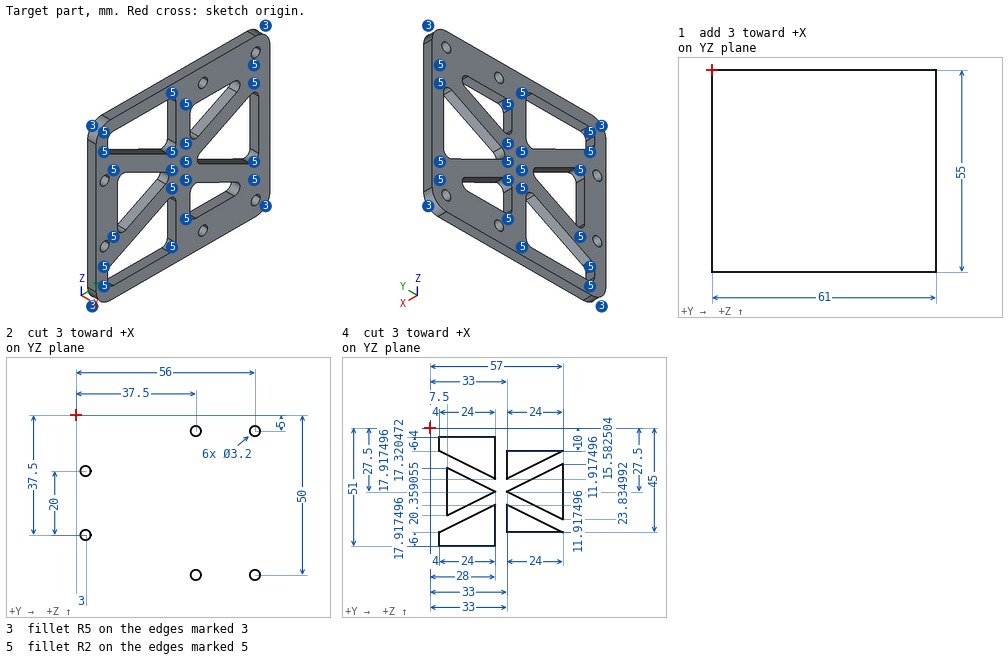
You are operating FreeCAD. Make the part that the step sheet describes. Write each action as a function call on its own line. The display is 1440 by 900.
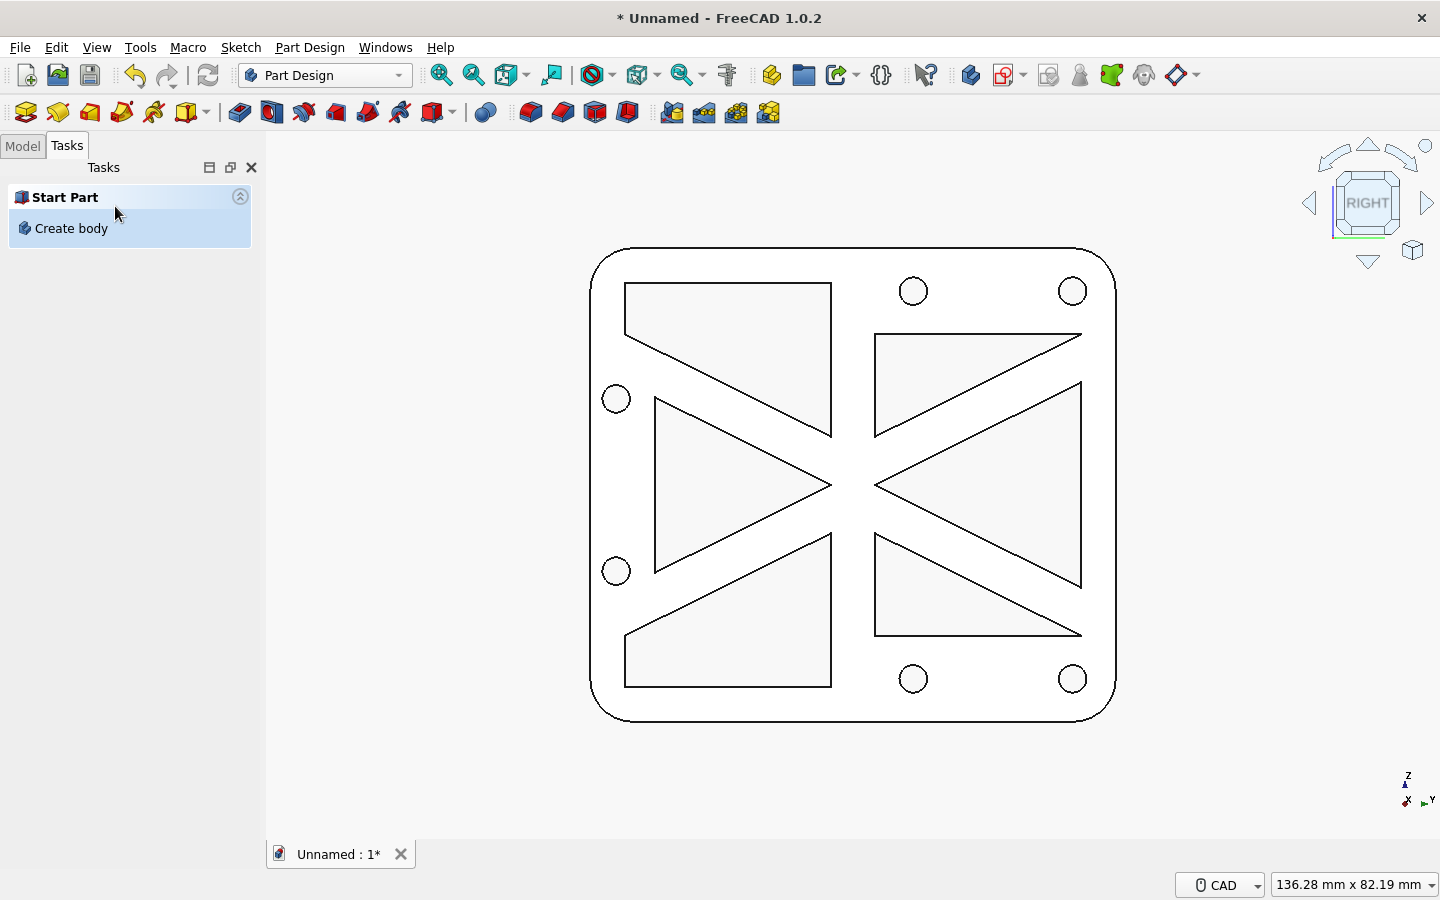
key(5)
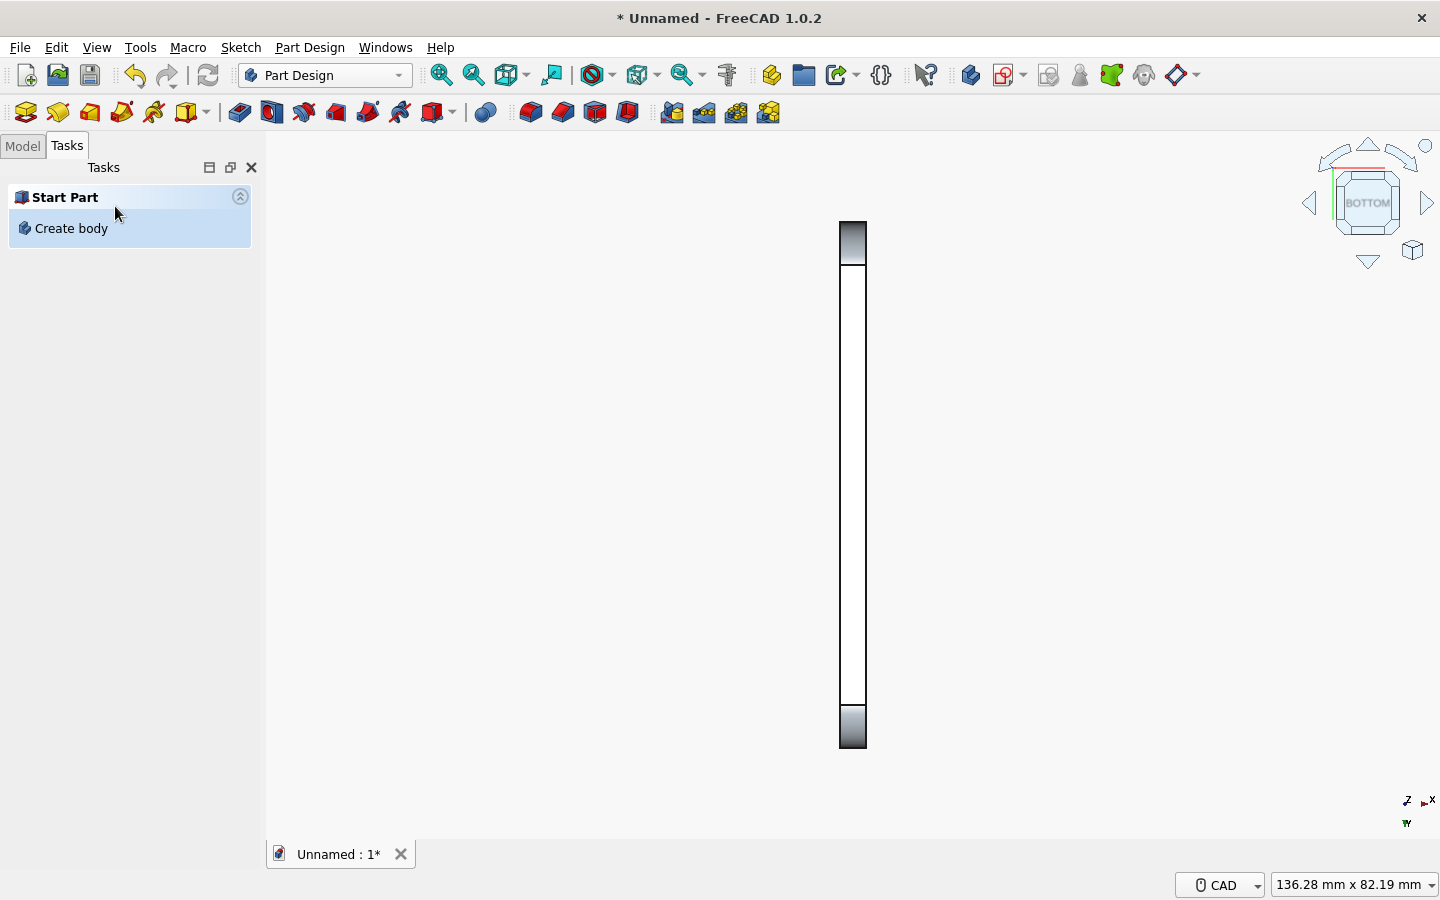
key(4)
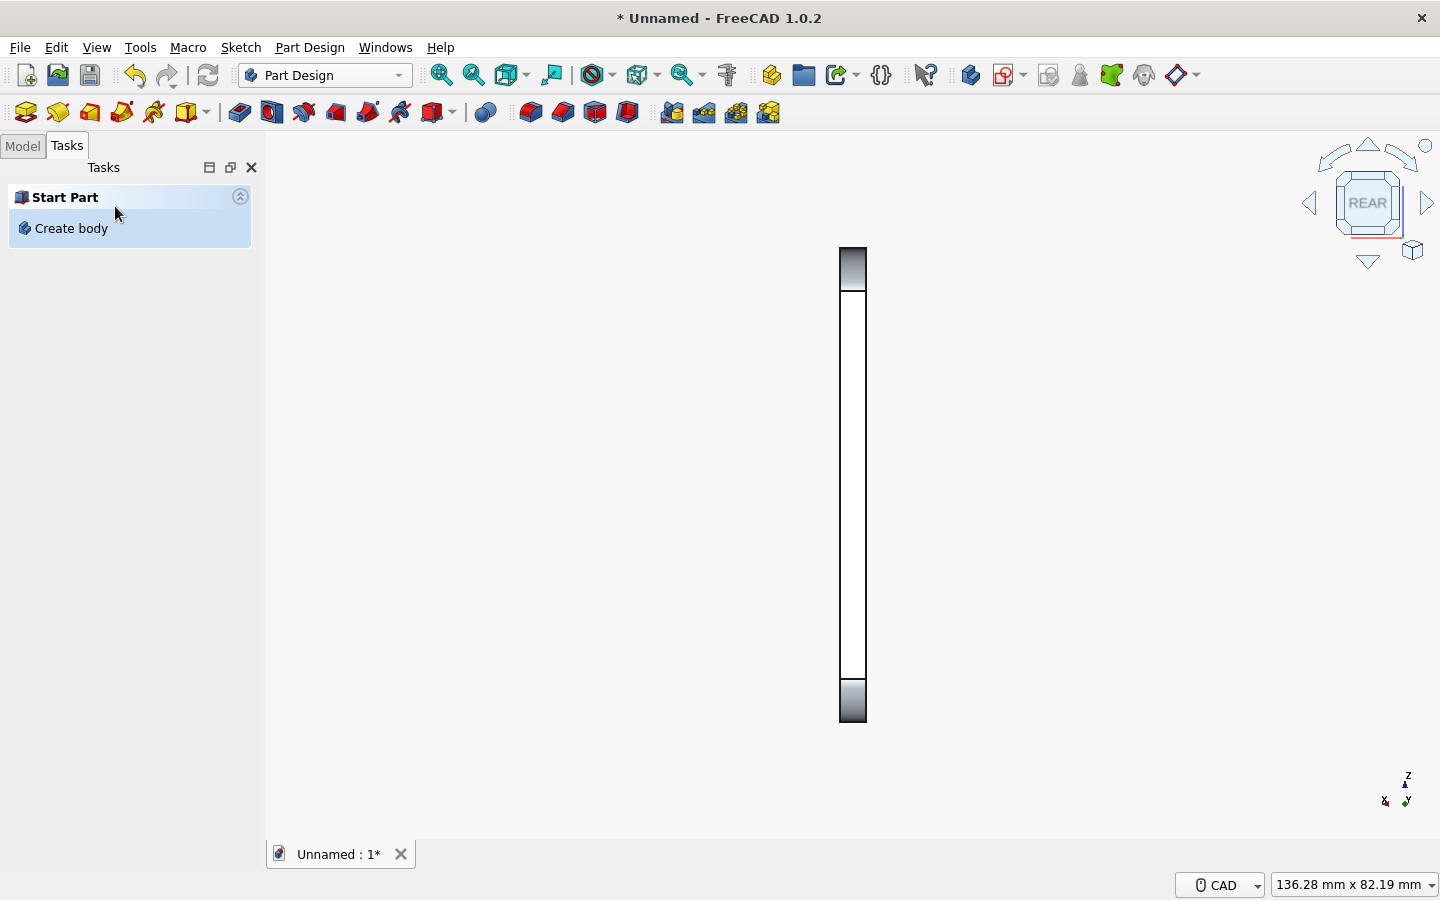
key(6)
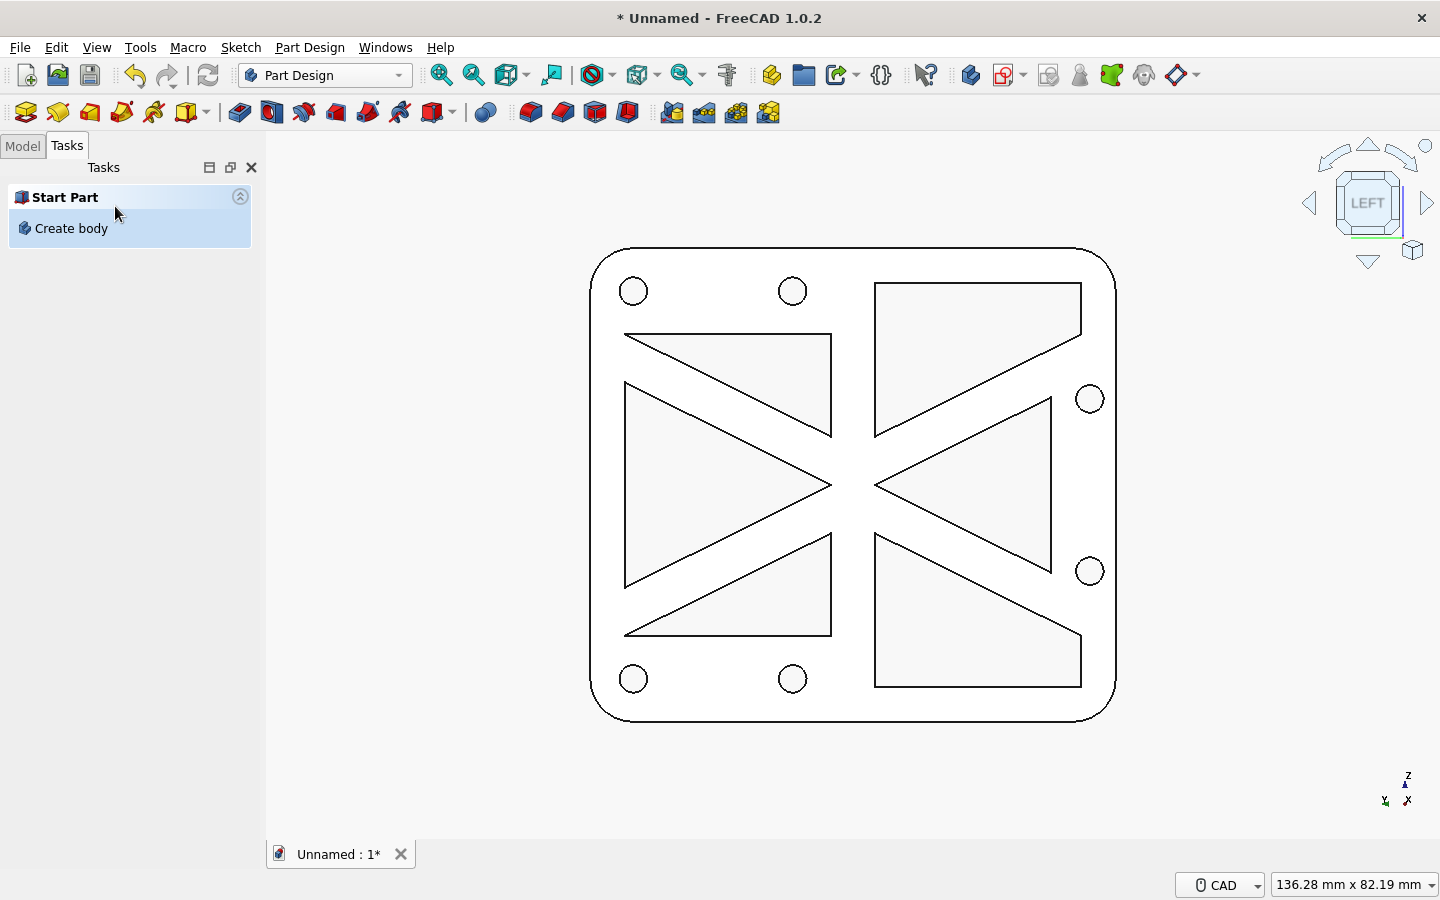
key(v)
key(3)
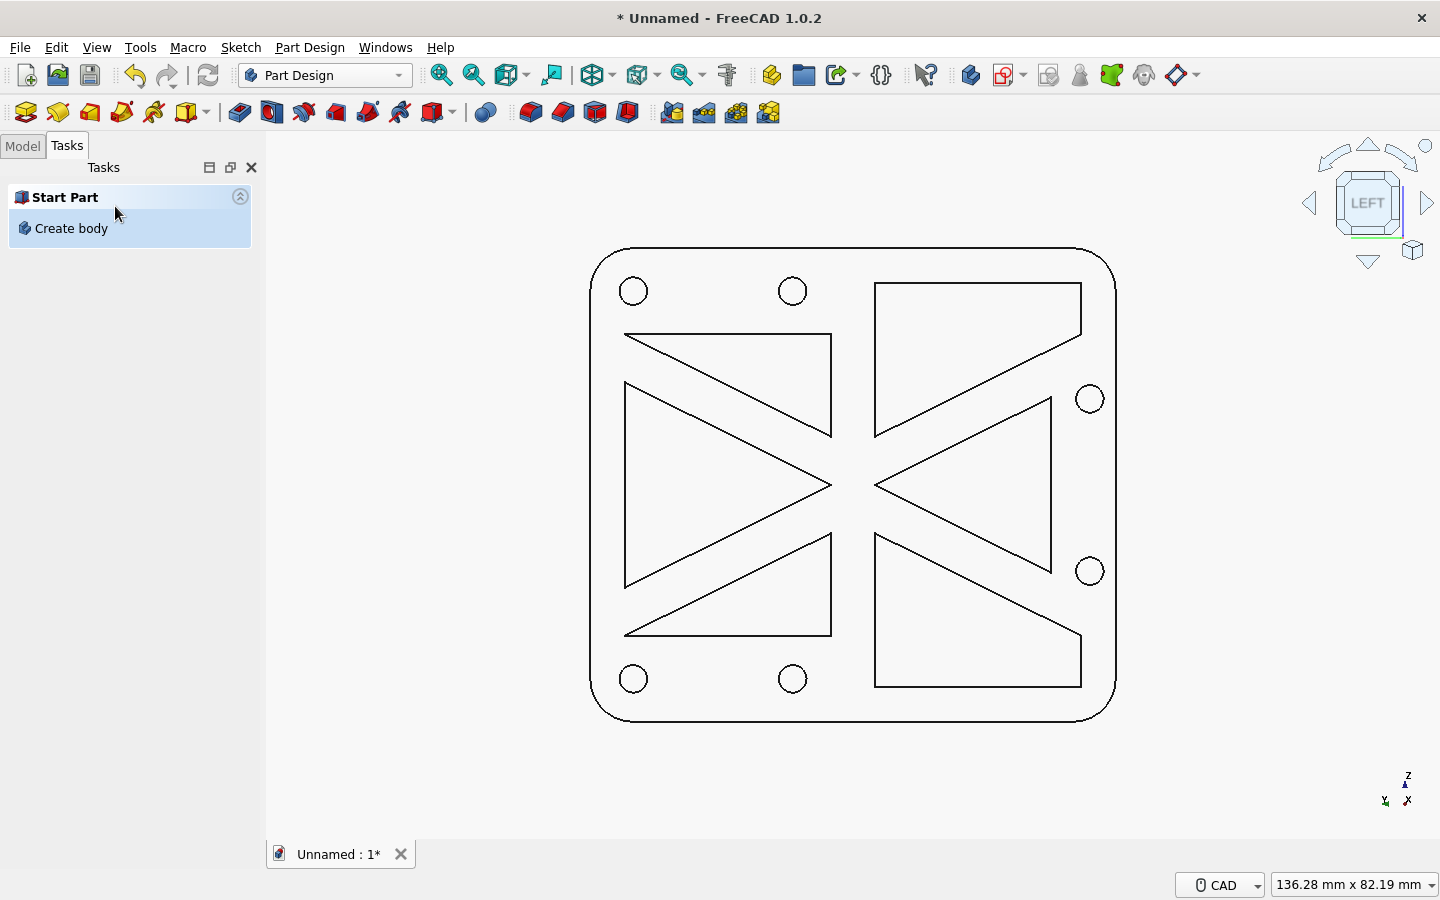
key(0)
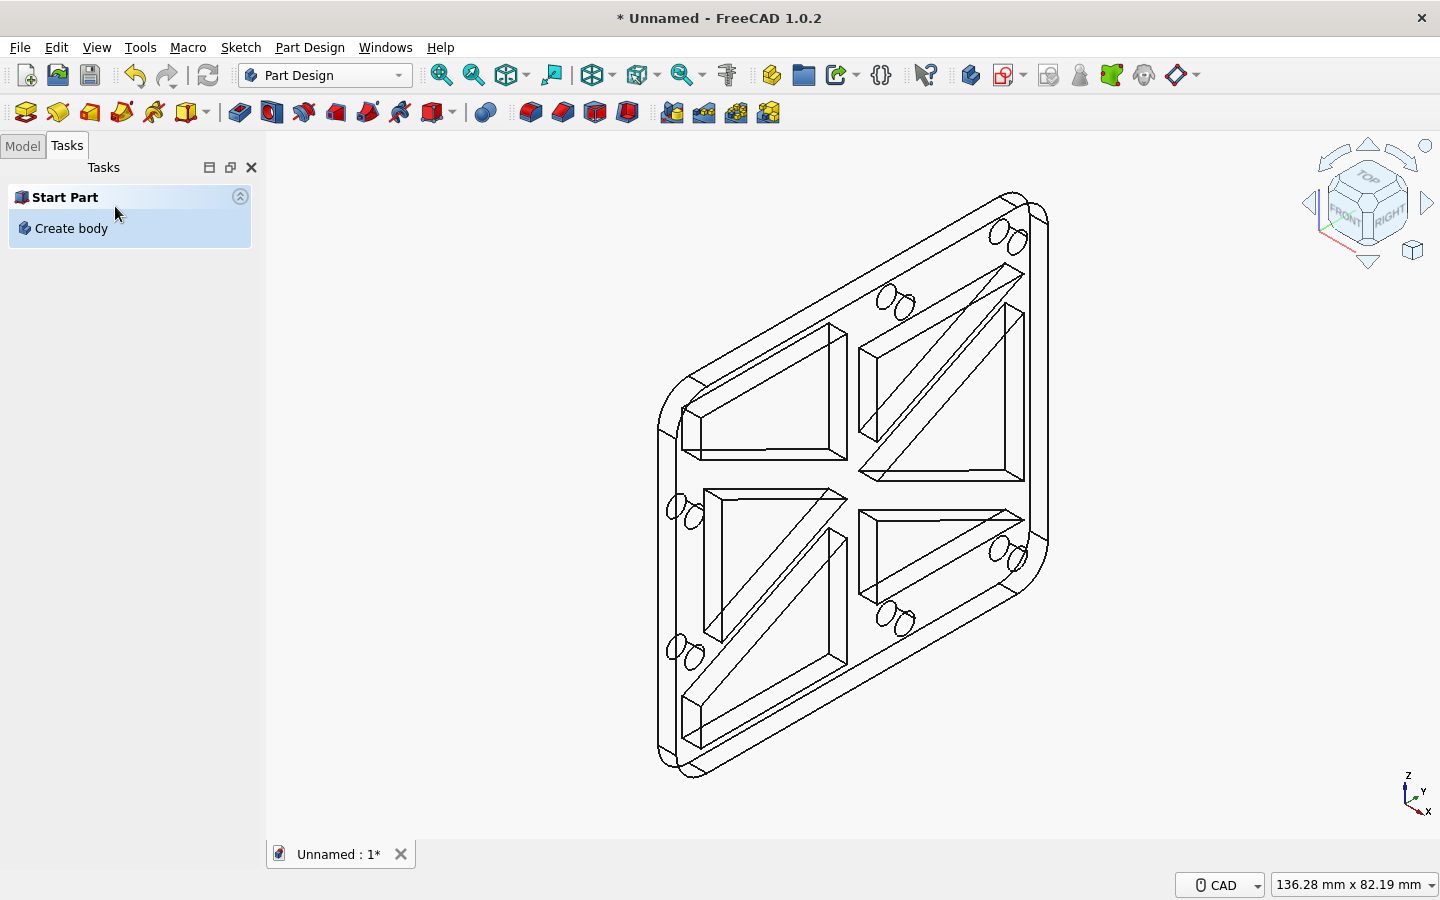
click(1013, 513)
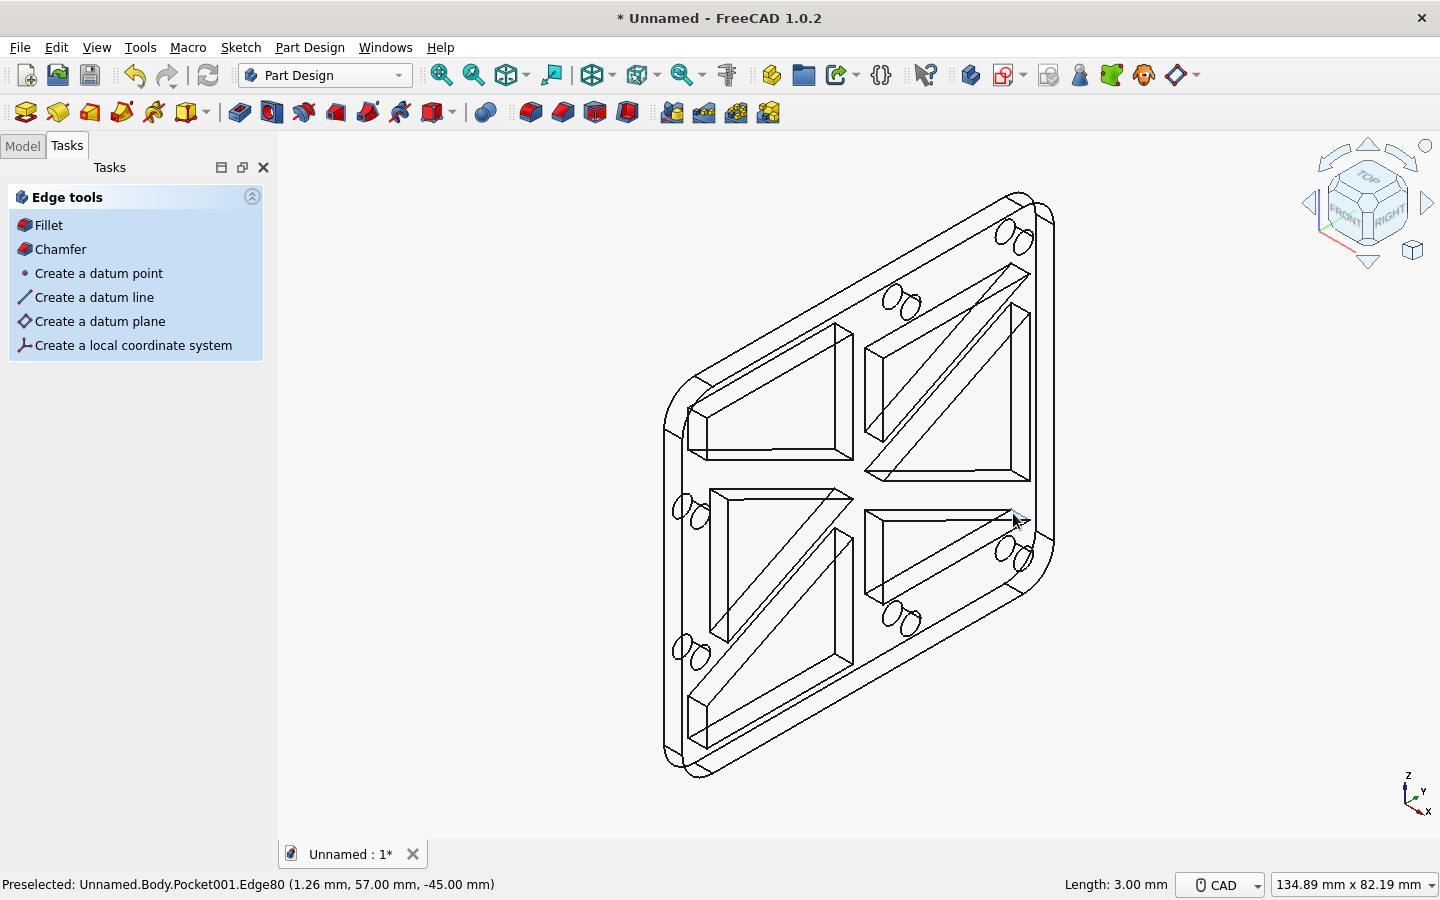
click(874, 514, ctrl)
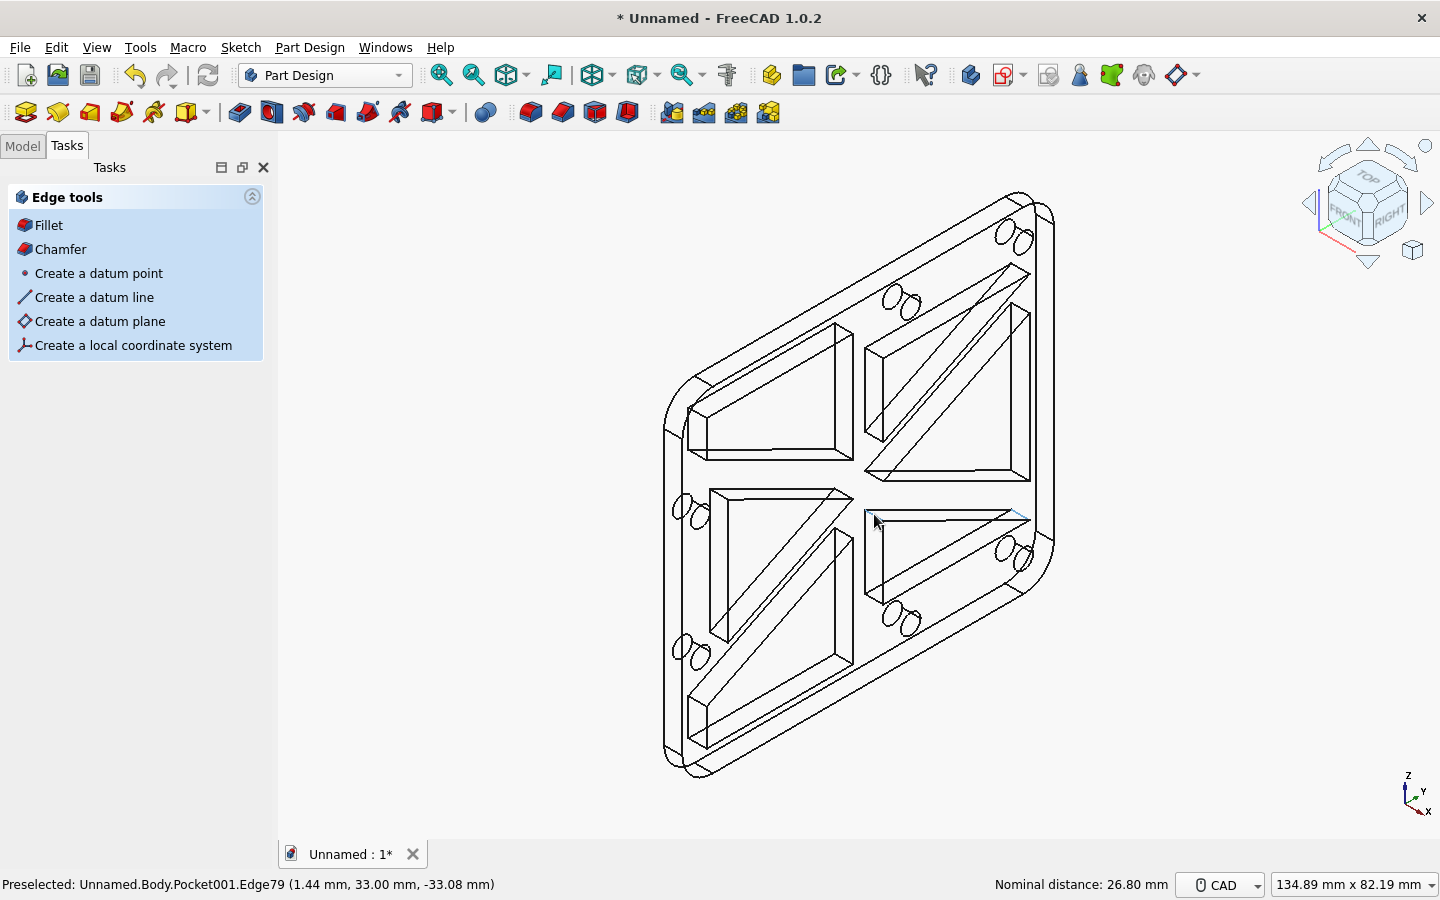
click(874, 598, ctrl)